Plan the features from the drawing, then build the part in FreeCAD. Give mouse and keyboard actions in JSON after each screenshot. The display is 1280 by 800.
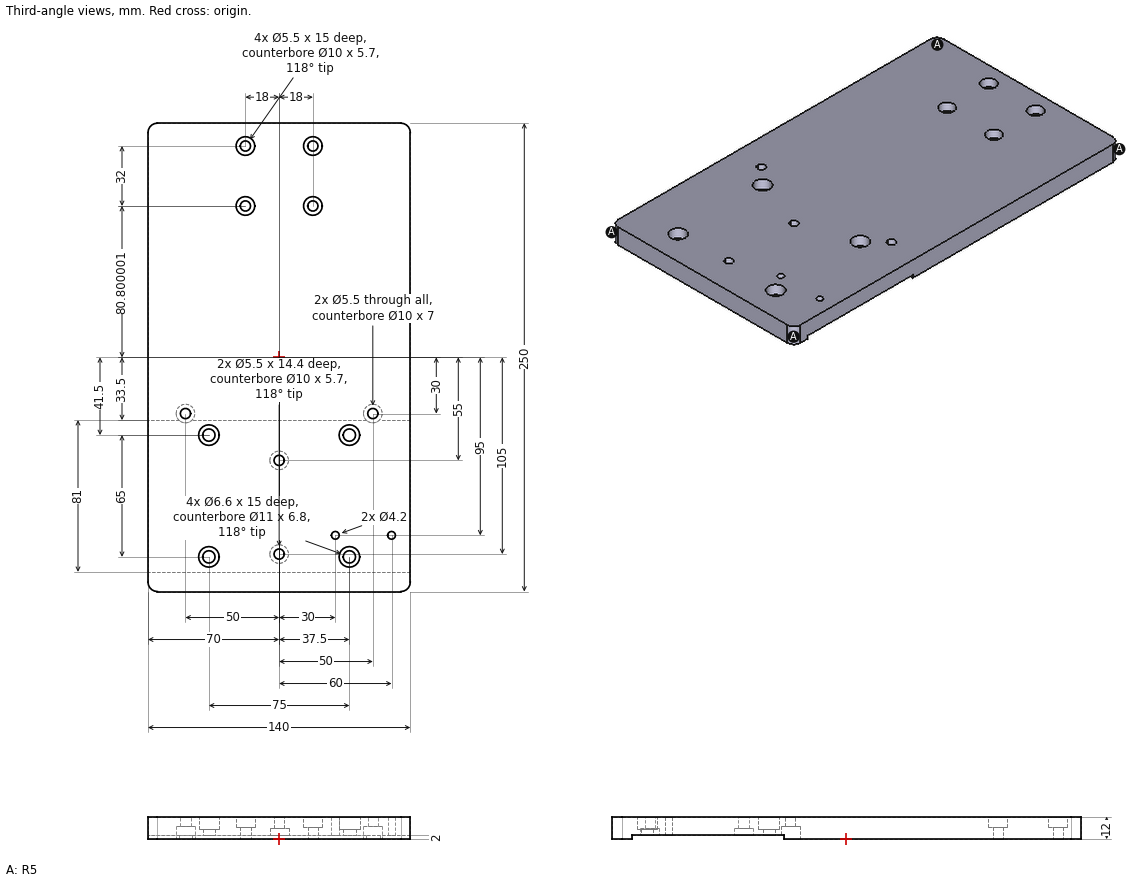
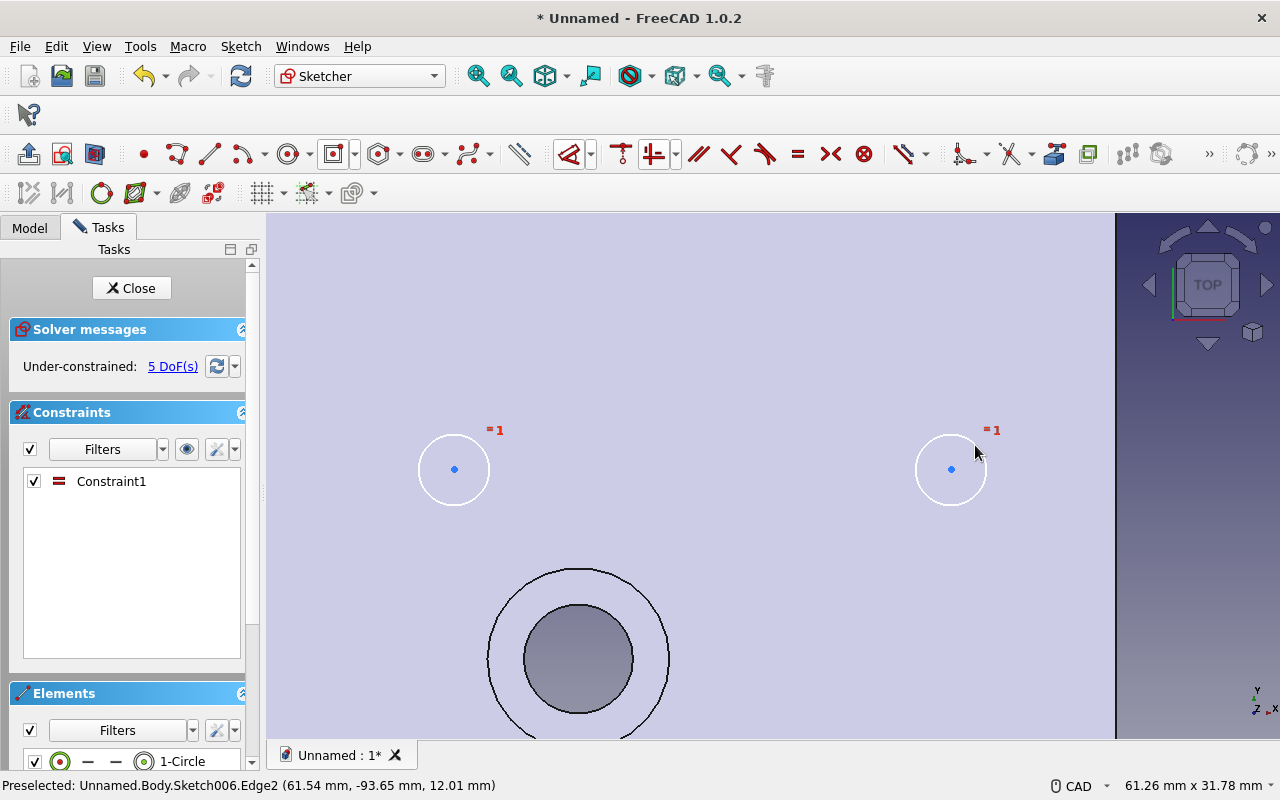
{"action": "left_click", "coordinate": [454, 470]}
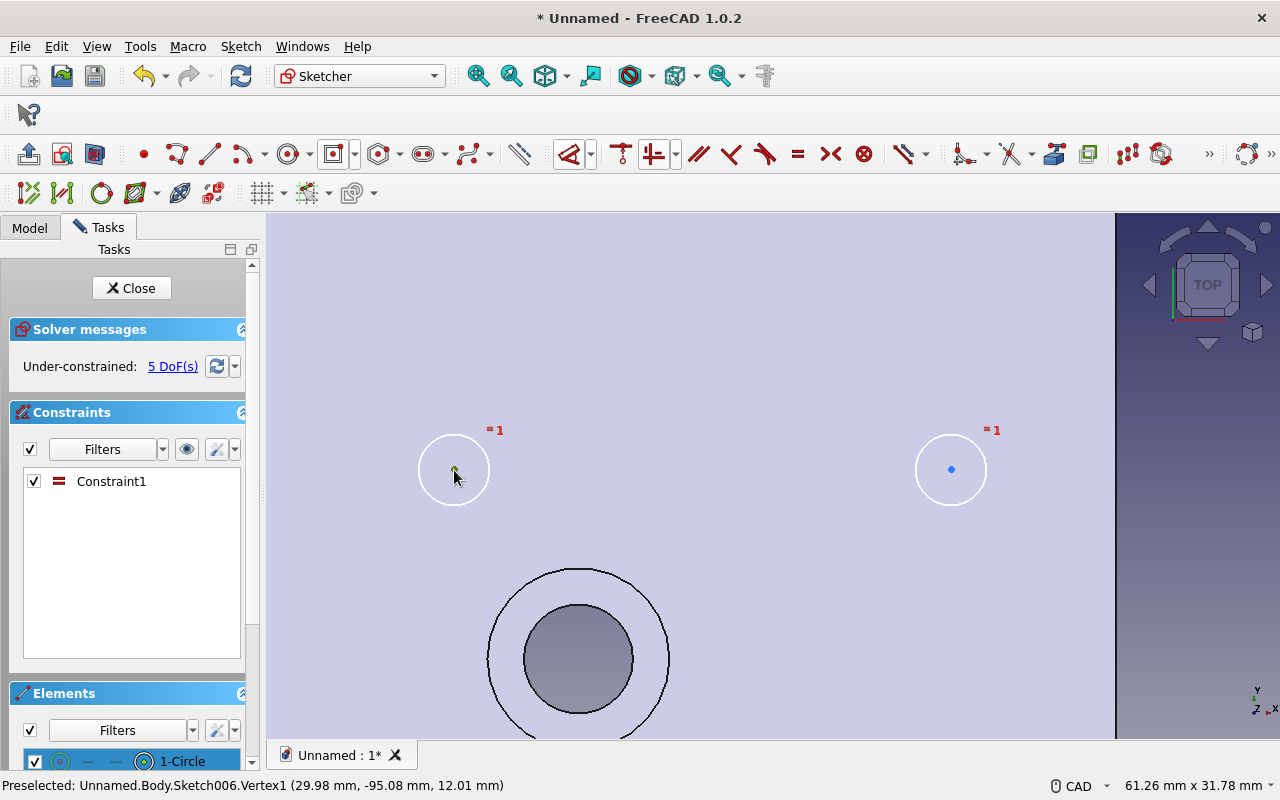
{"action": "left_click", "coordinate": [951, 470]}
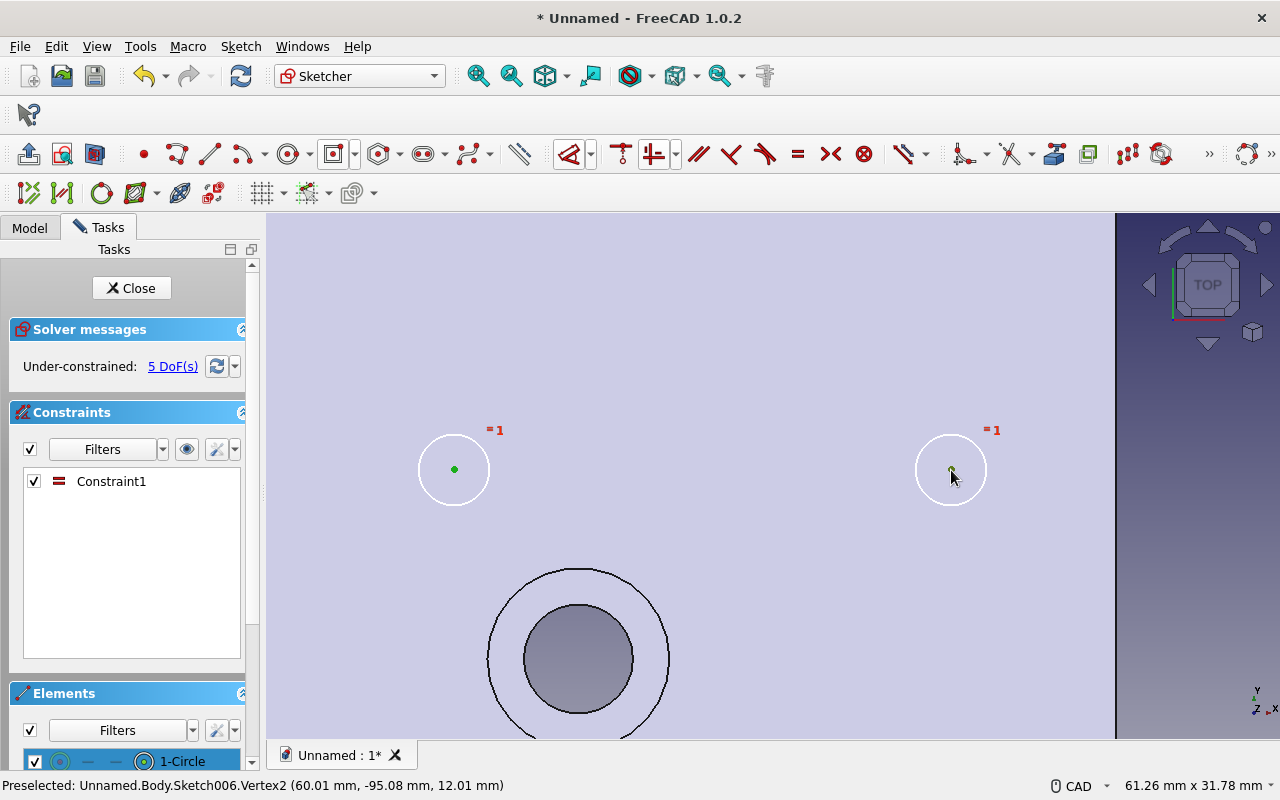
{"action": "key", "text": "h"}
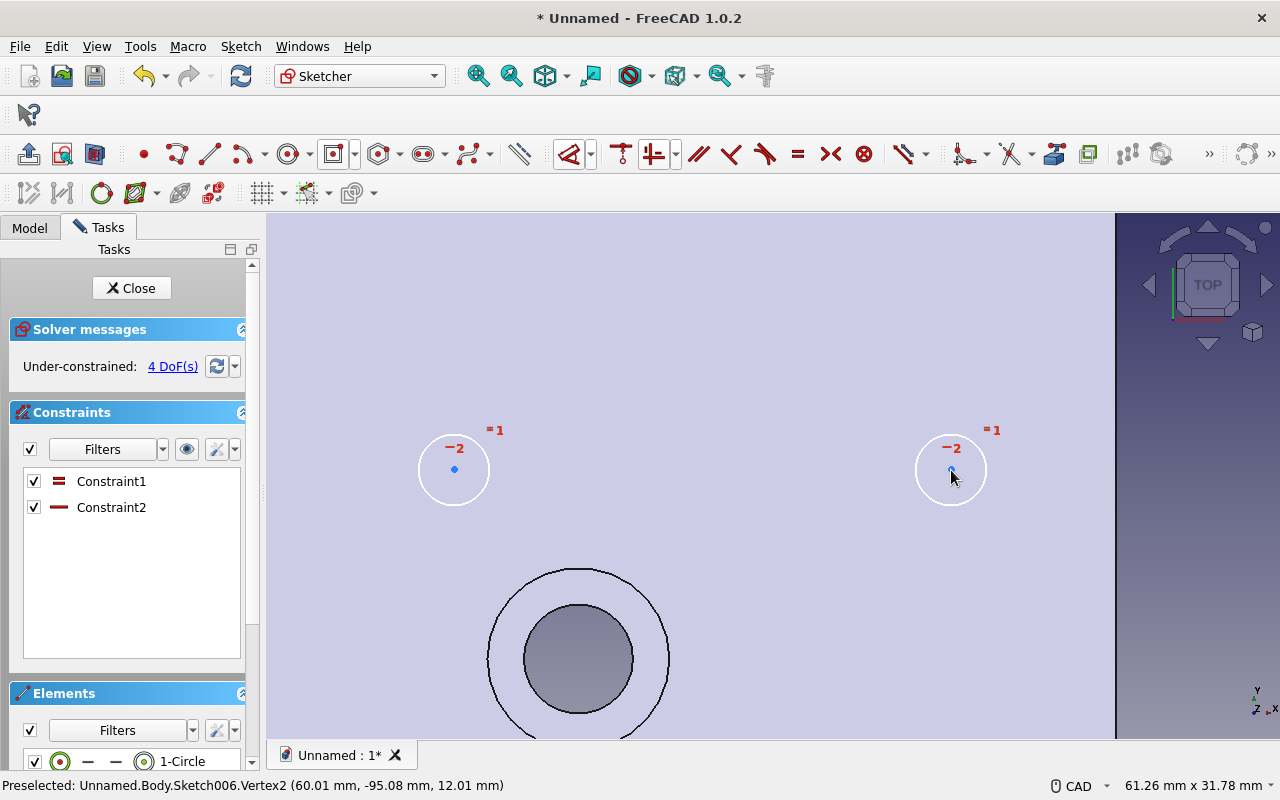
{"action": "left_click", "coordinate": [479, 445]}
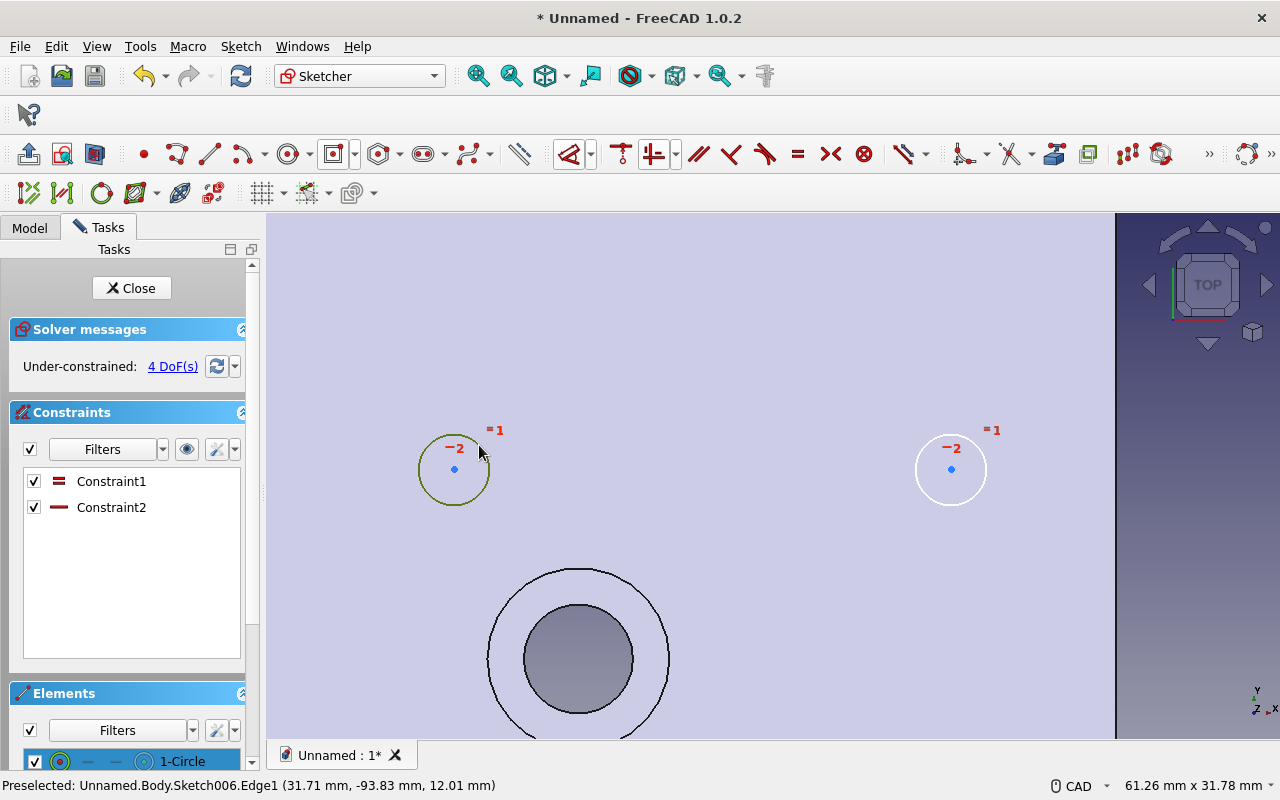
{"action": "key", "text": "k o"}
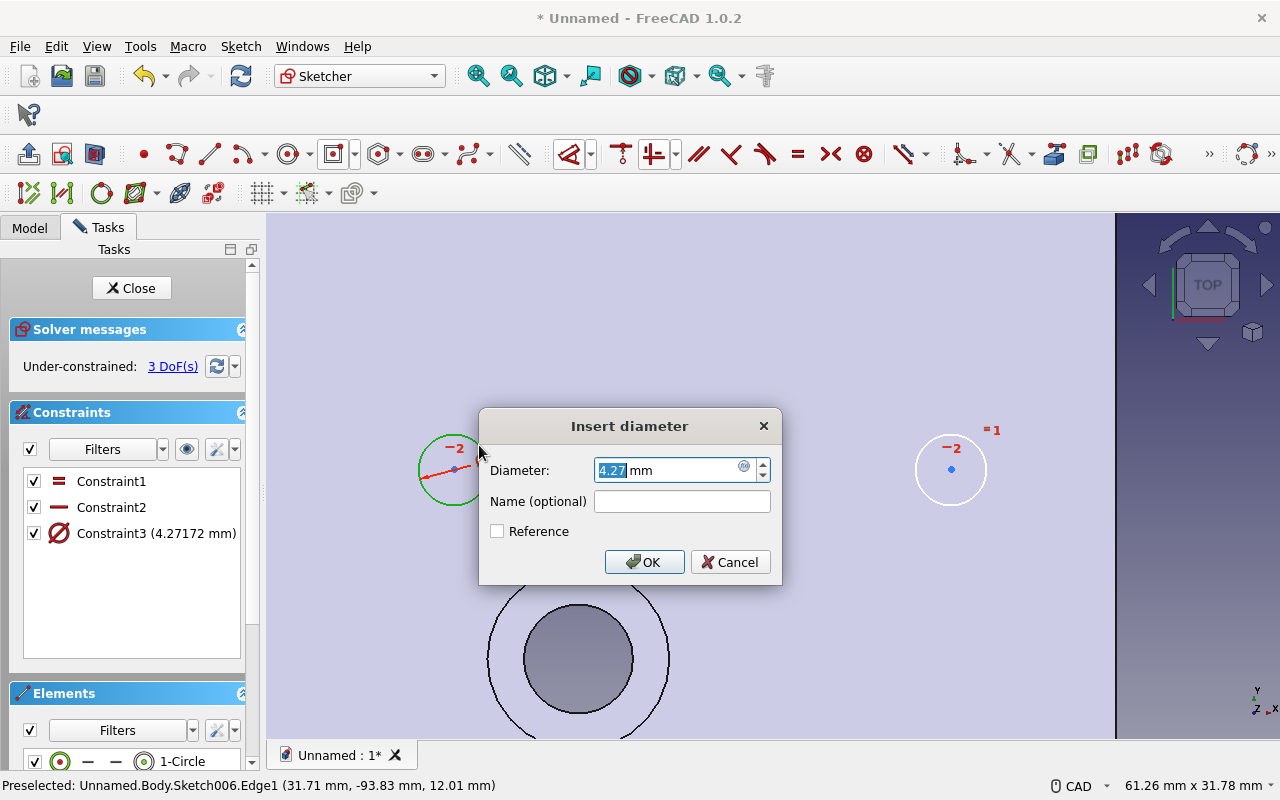
{"action": "type", "text": "4.2"}
{"action": "key", "text": "Return"}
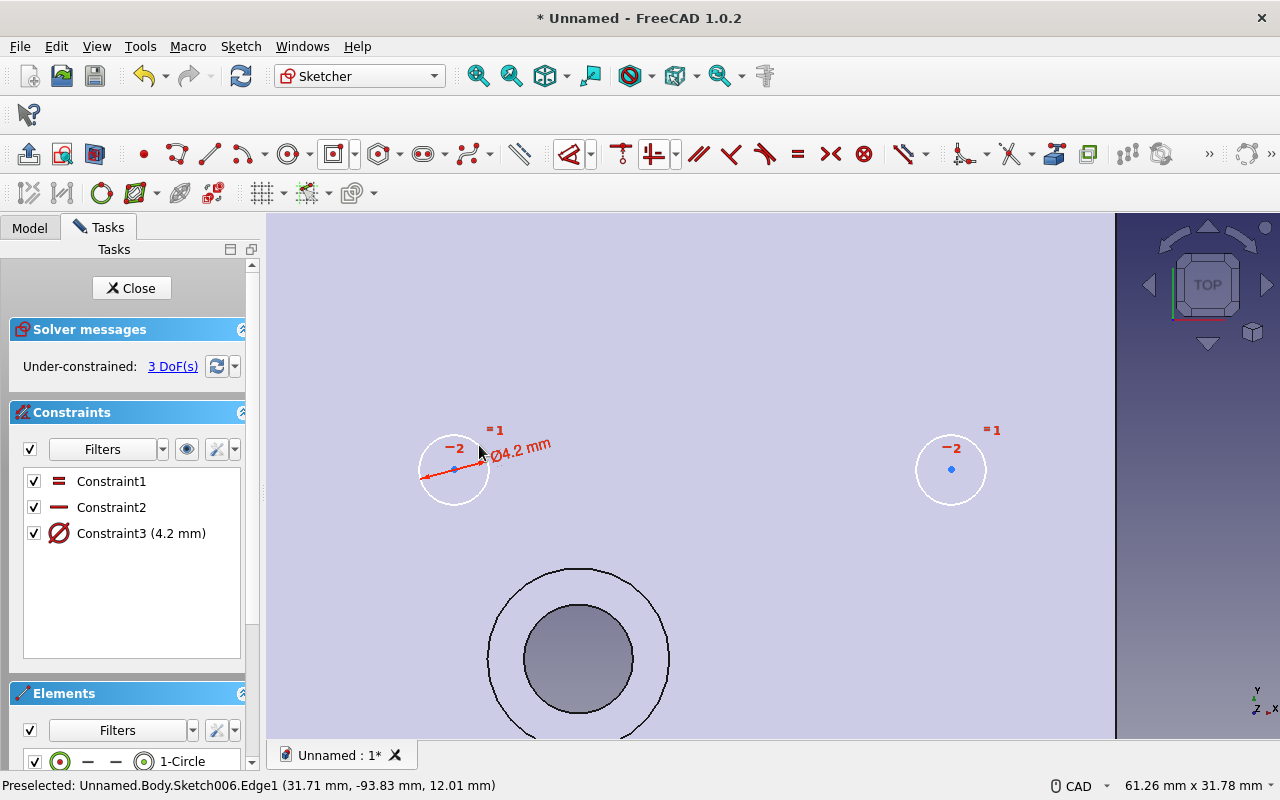
{"action": "left_click", "coordinate": [454, 470]}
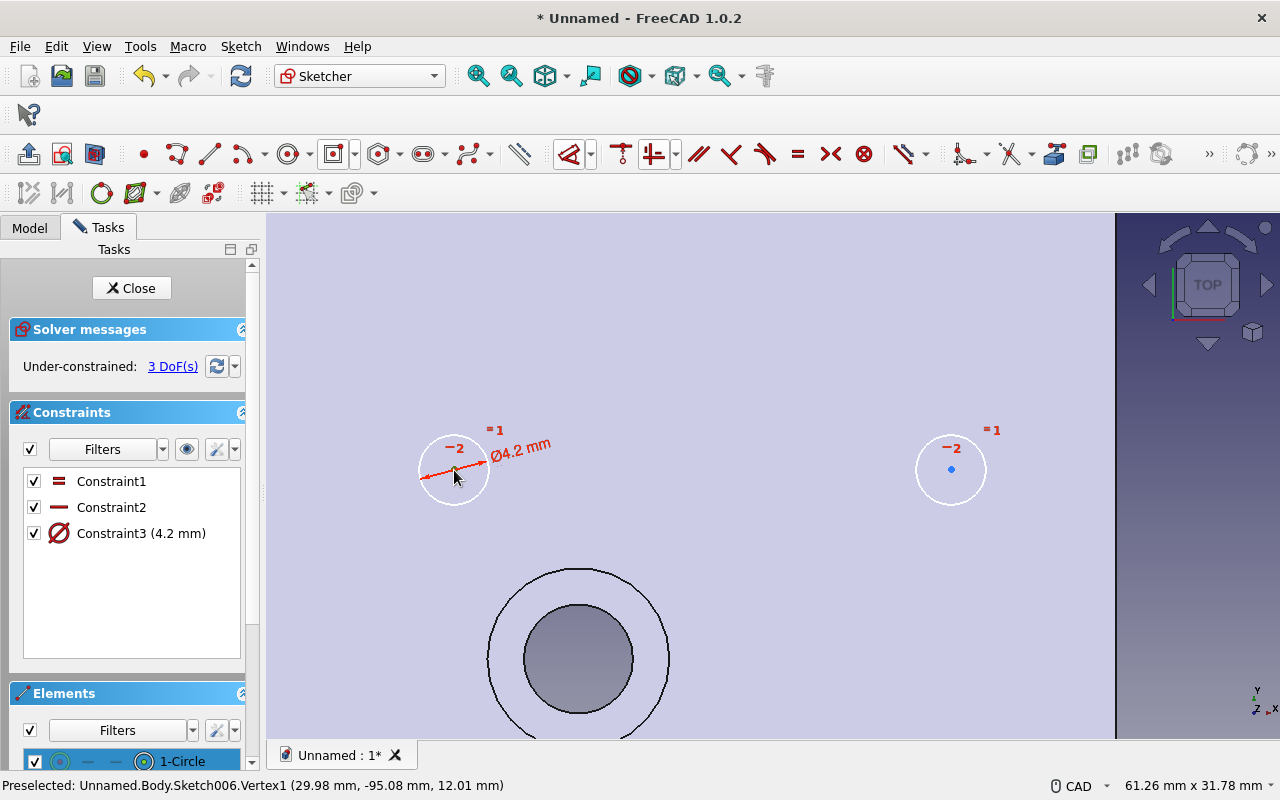
{"action": "key", "text": "l"}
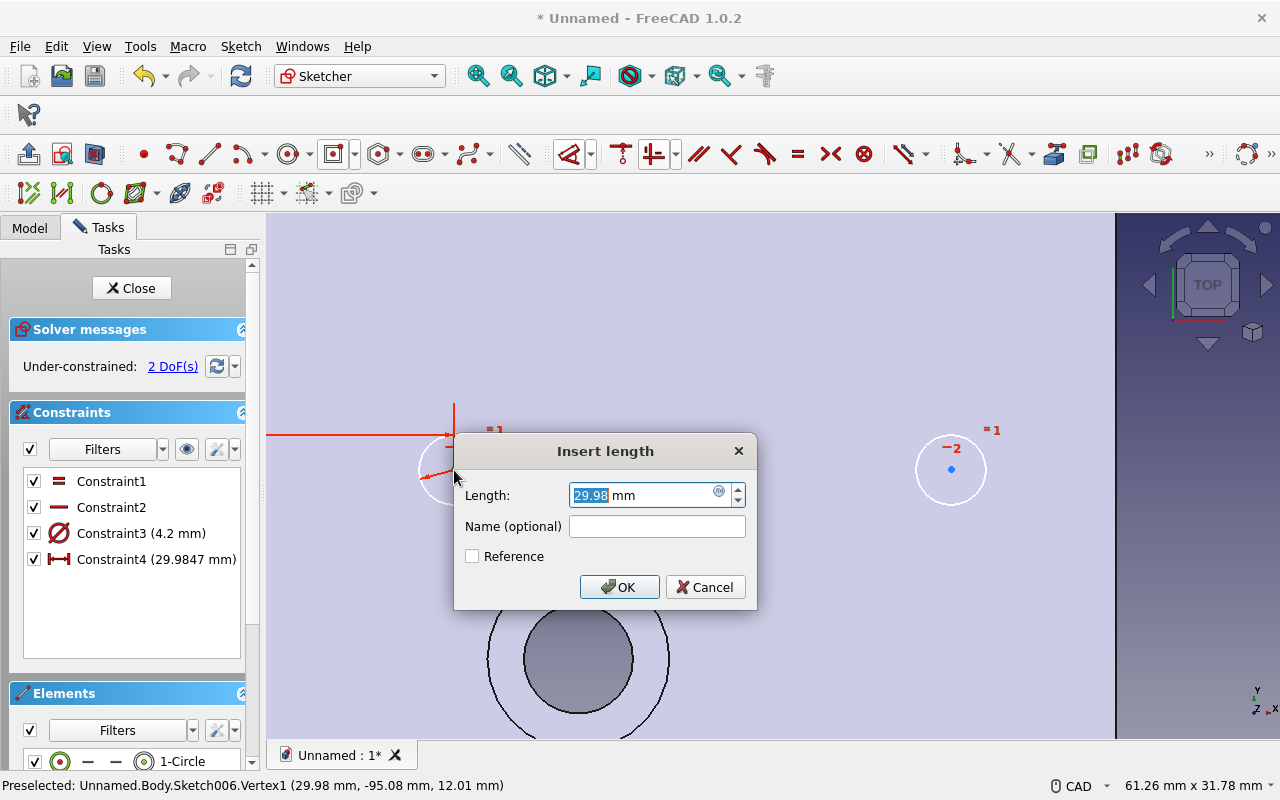
{"action": "type", "text": "30"}
{"action": "key", "text": "Return"}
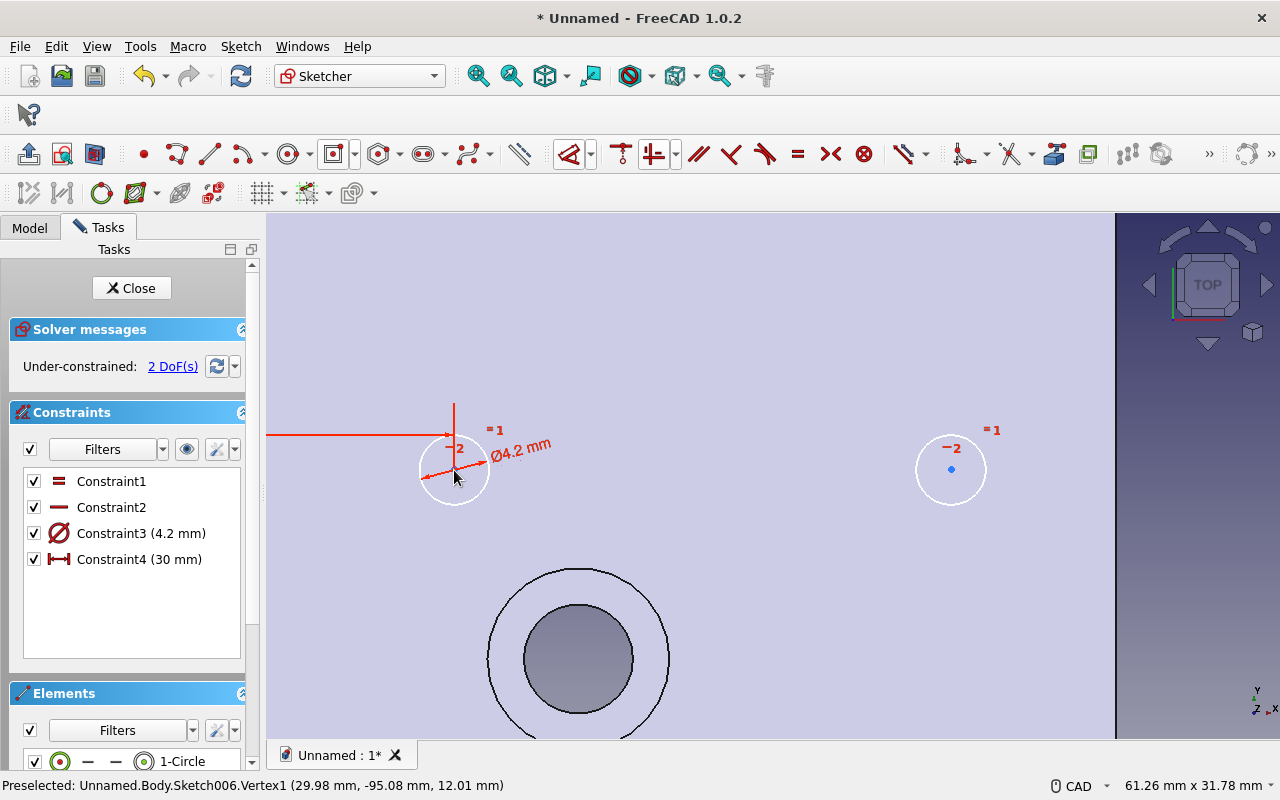
{"action": "left_click", "coordinate": [454, 470]}